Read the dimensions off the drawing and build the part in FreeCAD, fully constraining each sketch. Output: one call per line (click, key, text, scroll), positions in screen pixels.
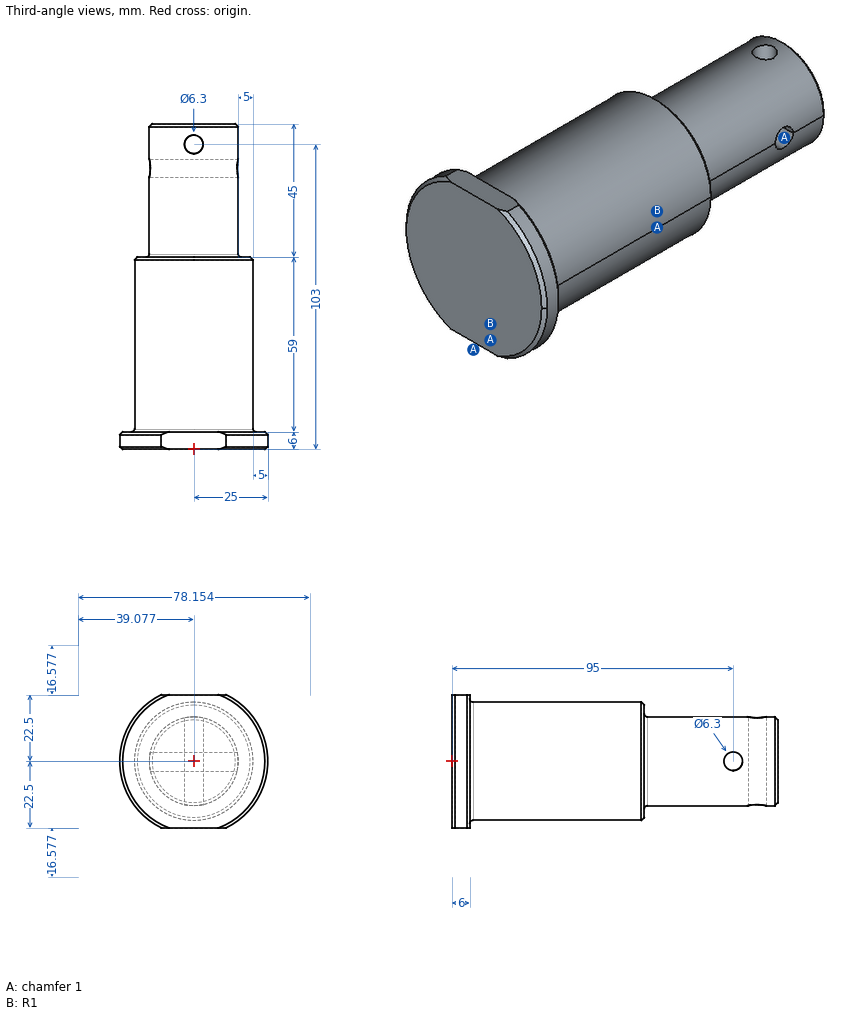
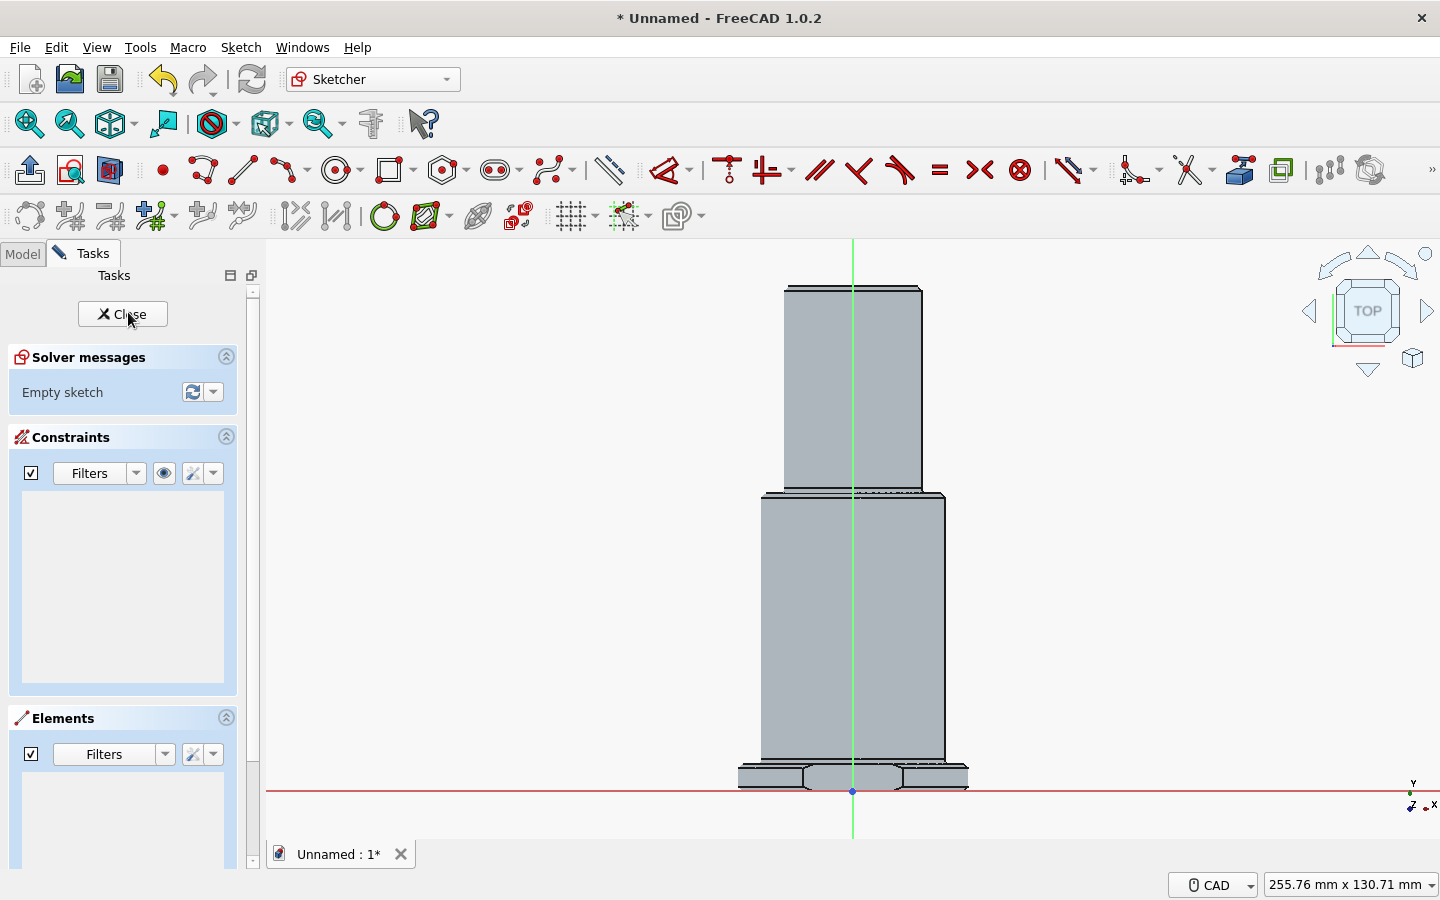
scroll(858, 301, up, 13)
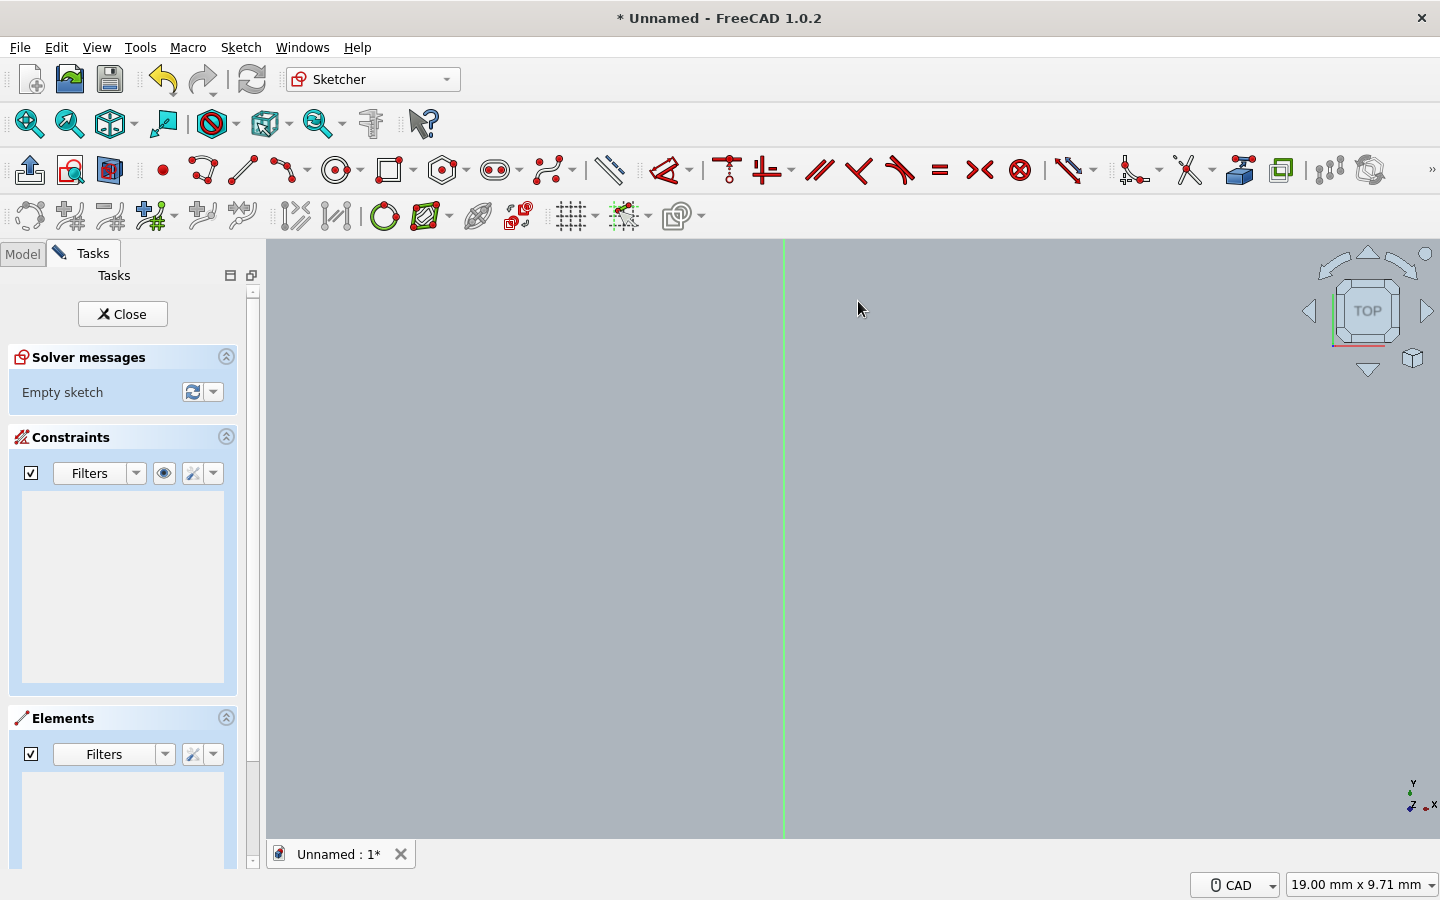
key(g)
key(c)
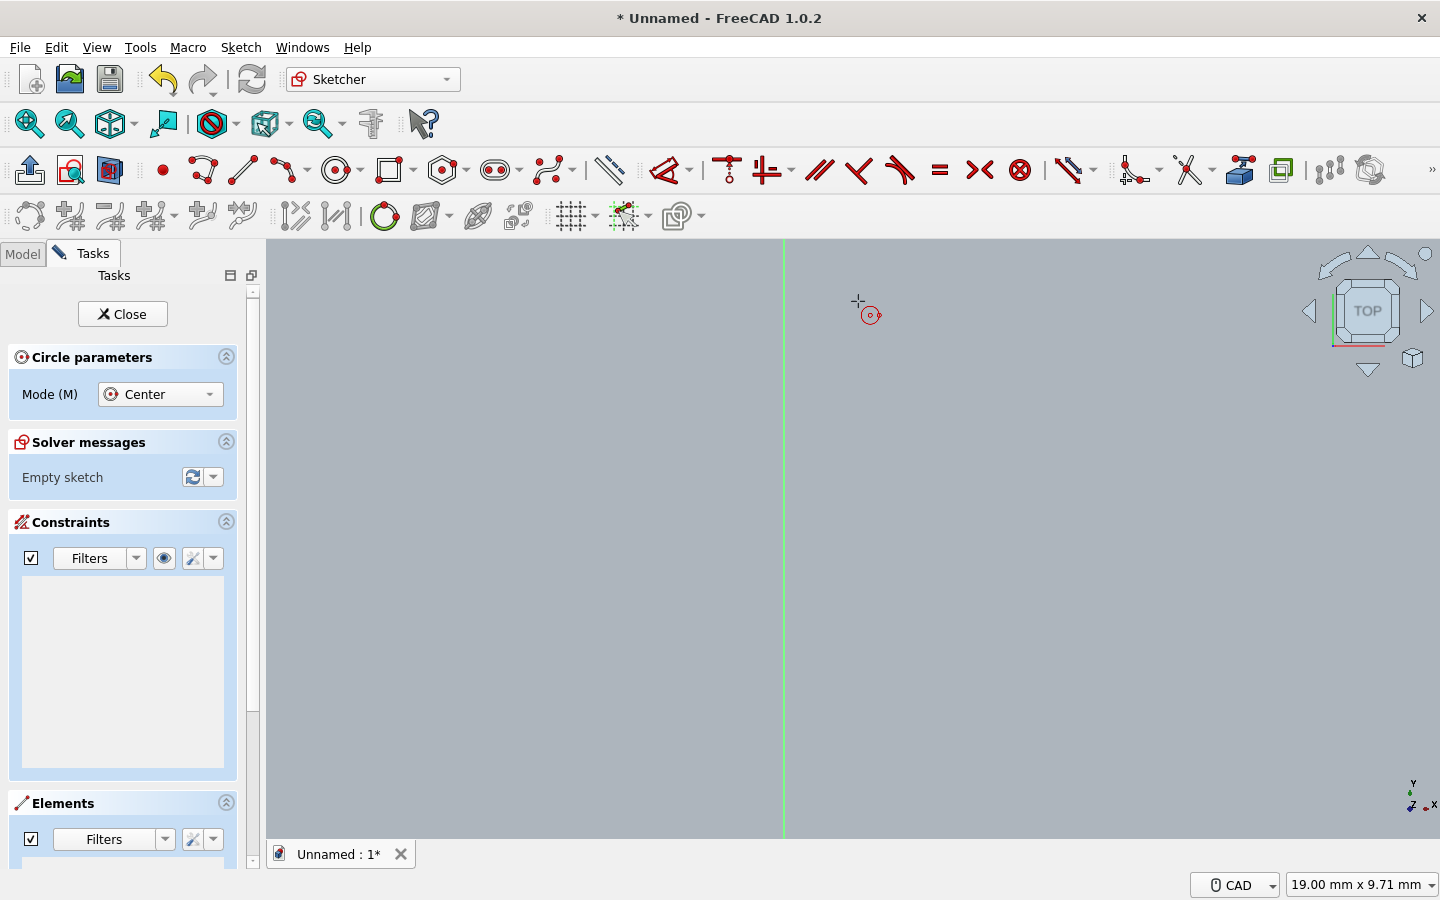
click(784, 537)
click(921, 399)
key(Escape)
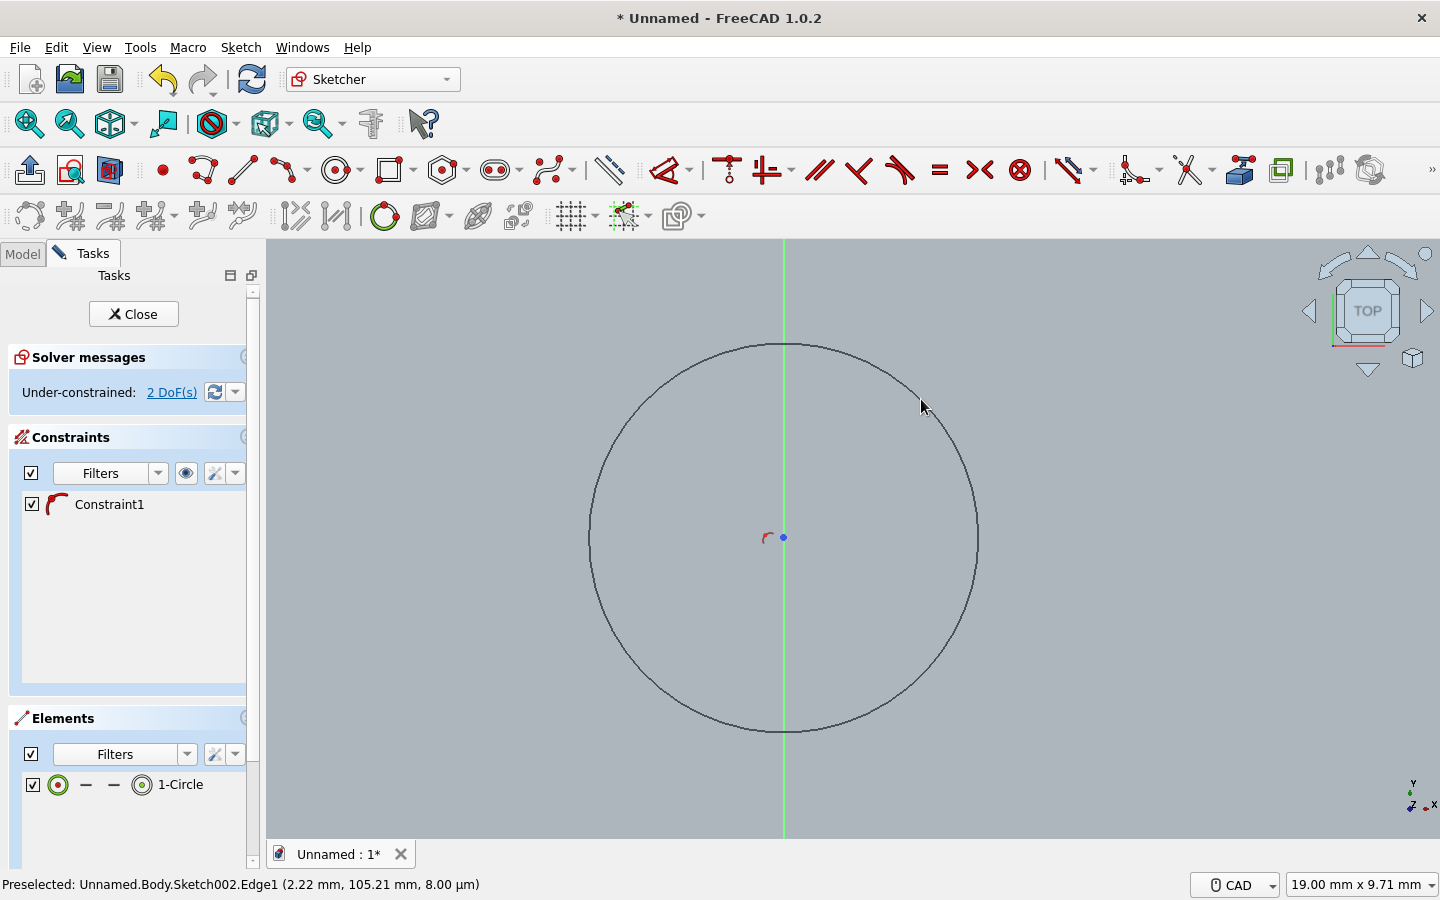
key(d)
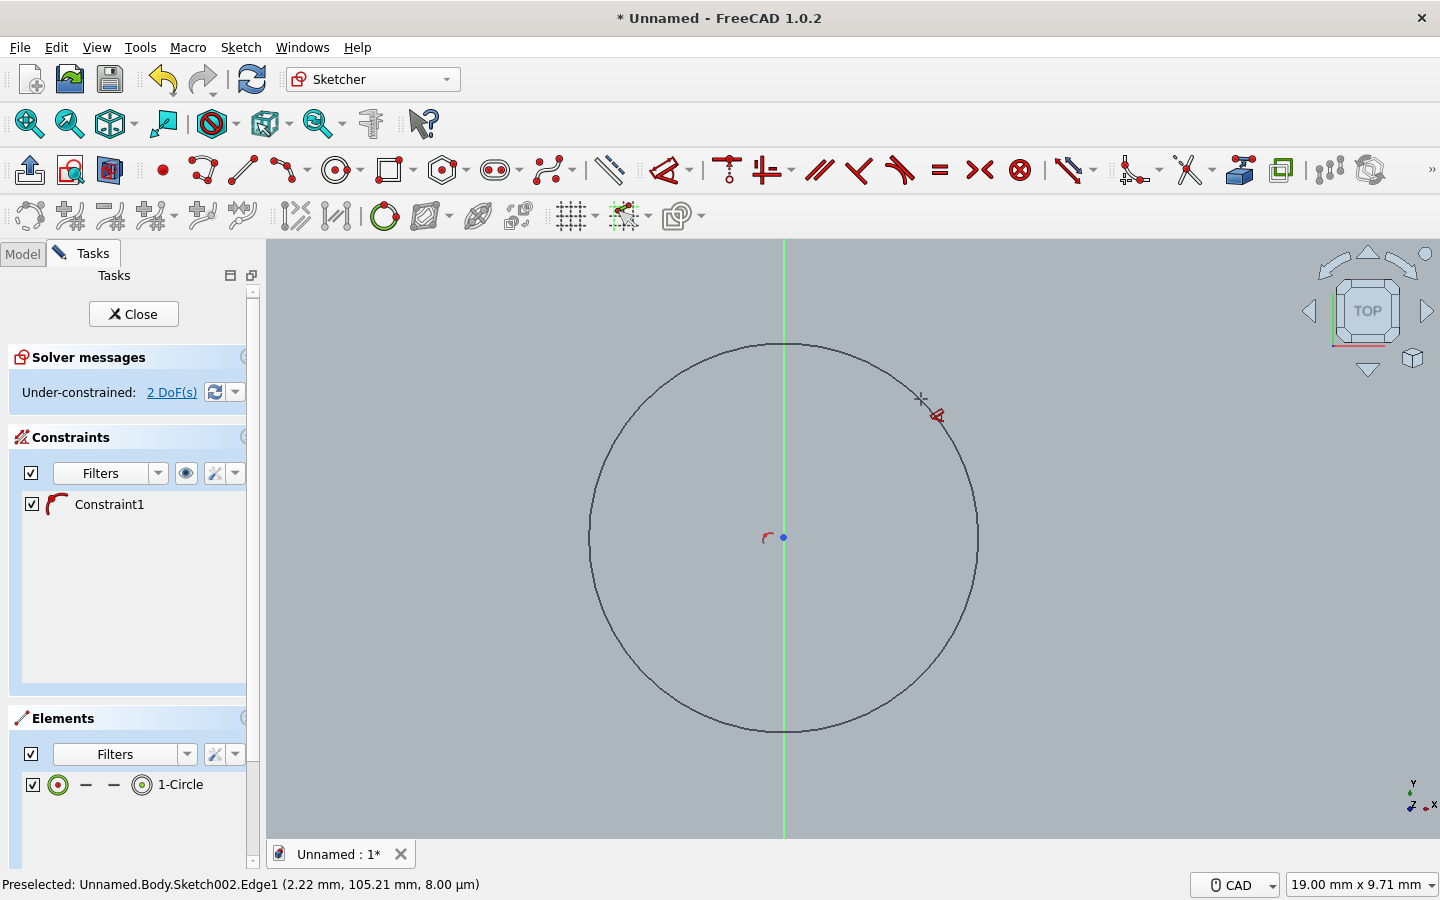
click(921, 400)
click(944, 377)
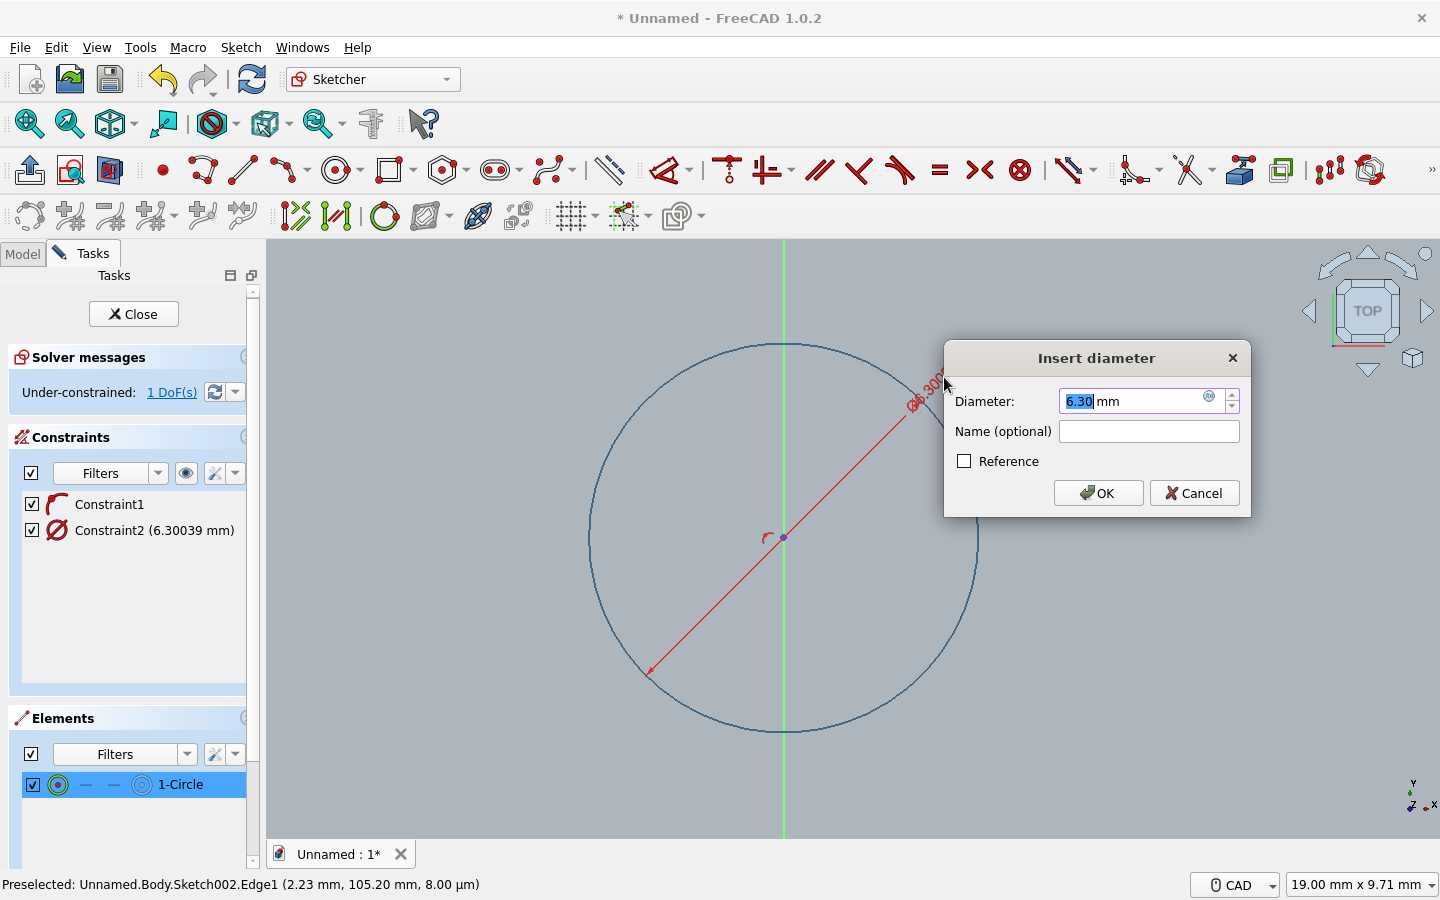
text(6.3)
key(Return)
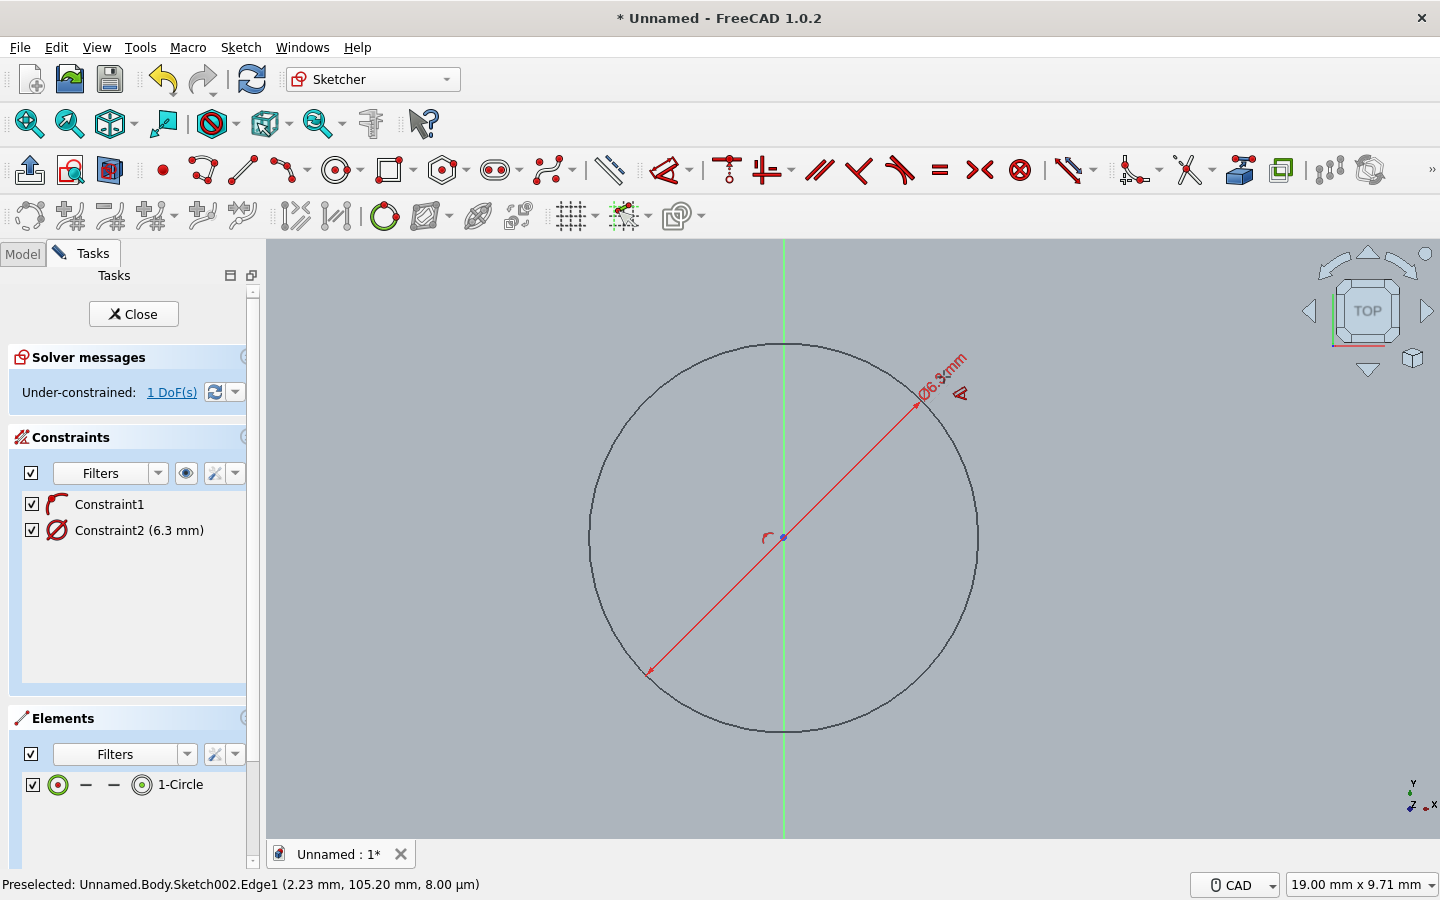
click(784, 538)
click(818, 674)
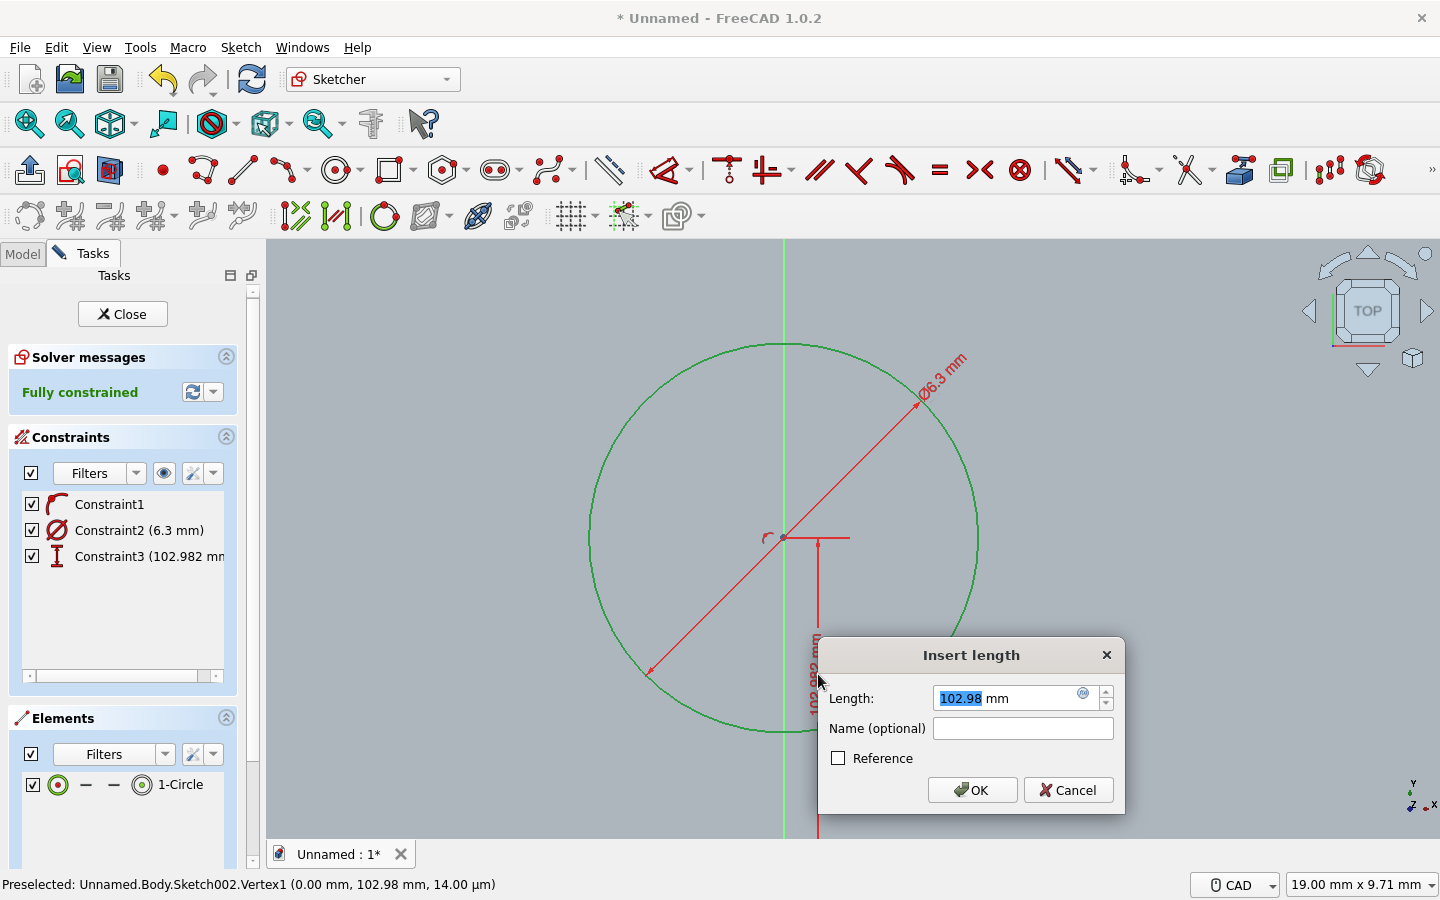
text(103)
key(Return)
key(Escape)